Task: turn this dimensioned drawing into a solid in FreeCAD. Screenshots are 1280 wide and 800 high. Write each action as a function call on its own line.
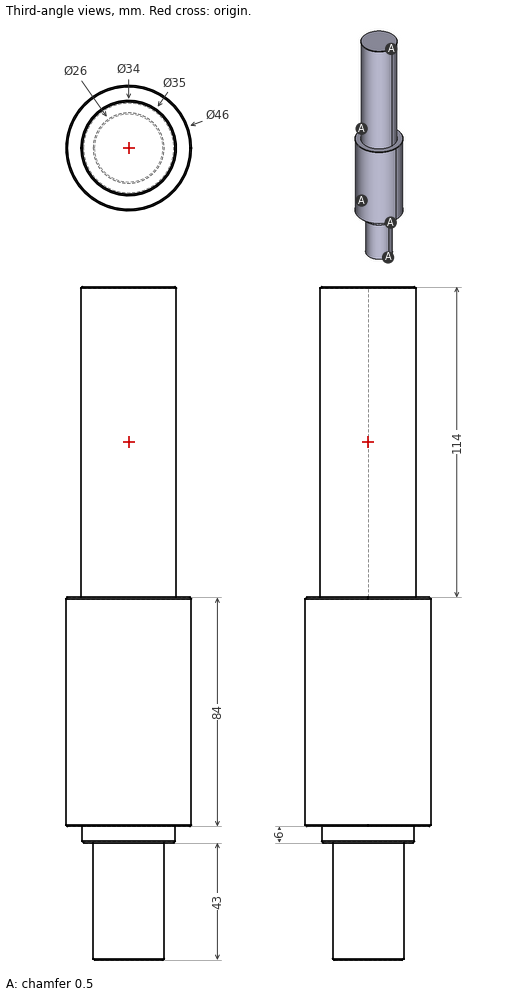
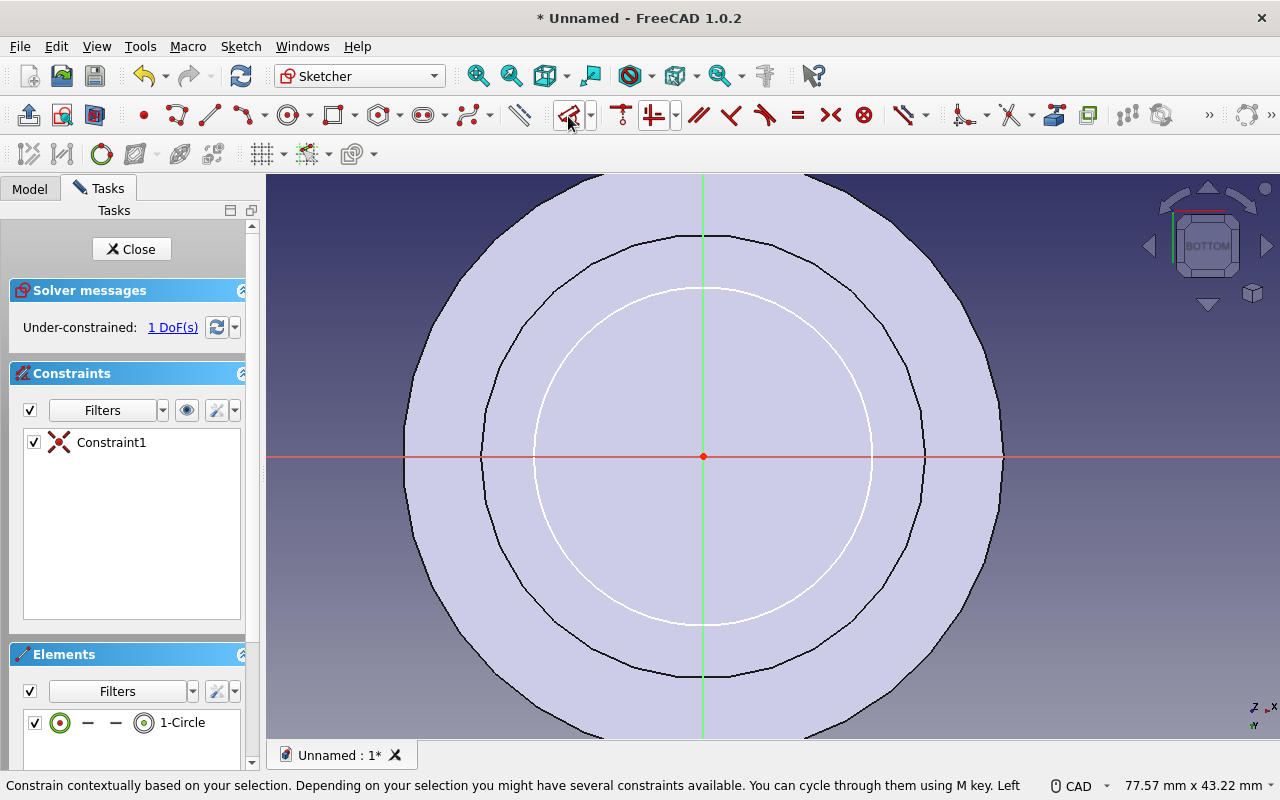
click(822, 336)
click(844, 313)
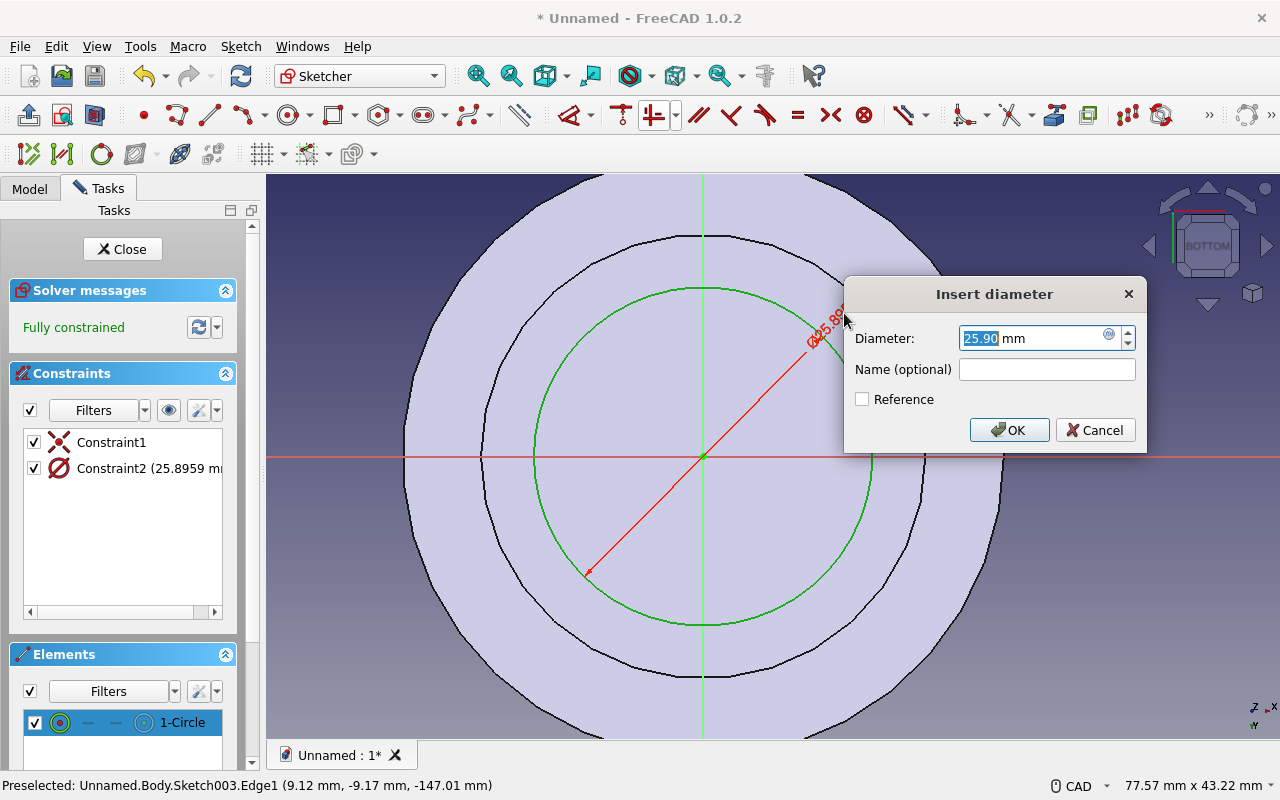
text(26)
key(Return)
key(Escape)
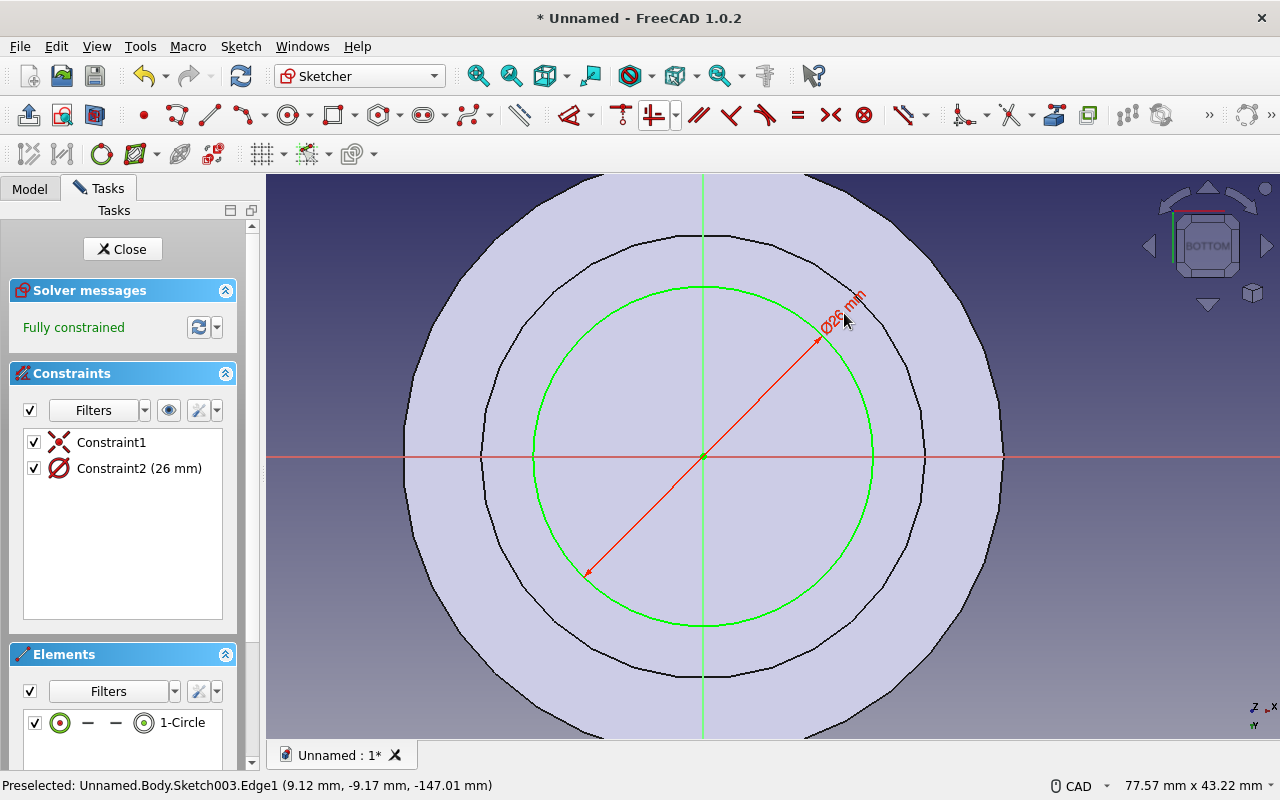
click(123, 249)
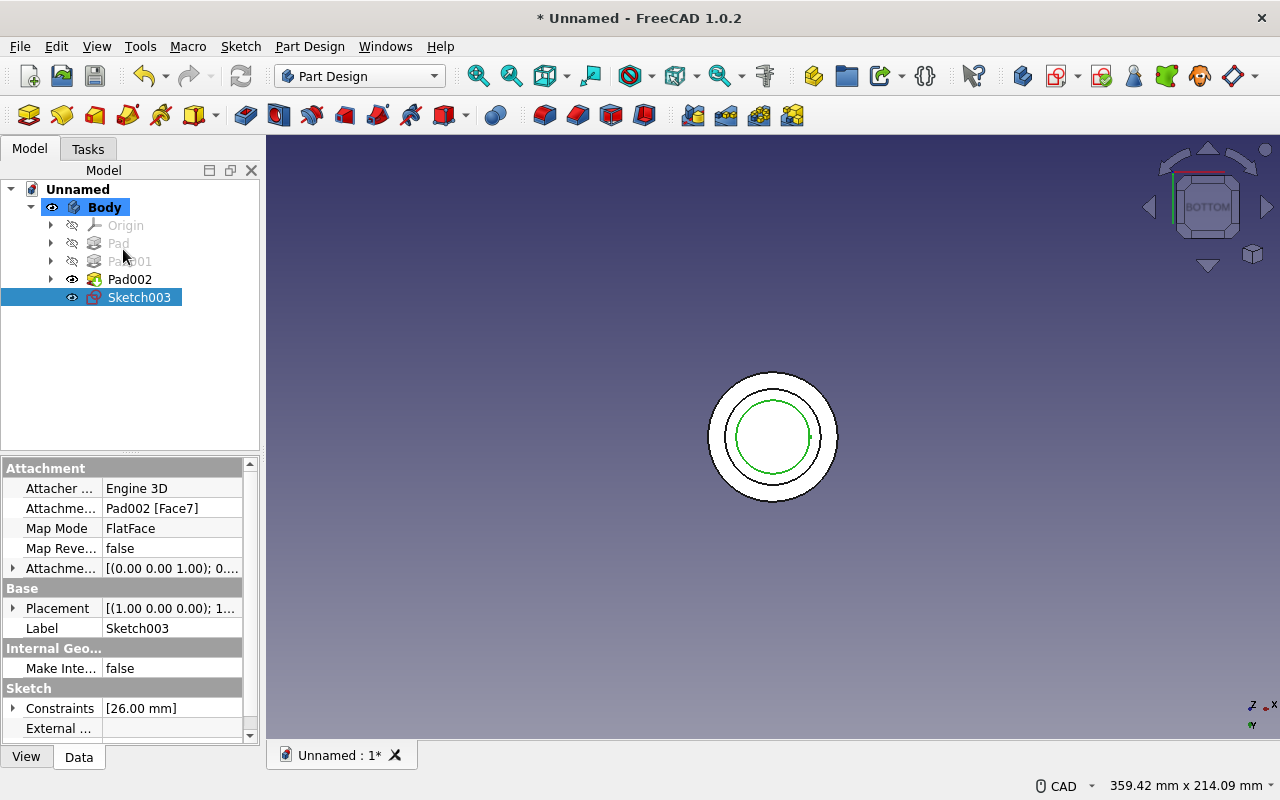
click(29, 116)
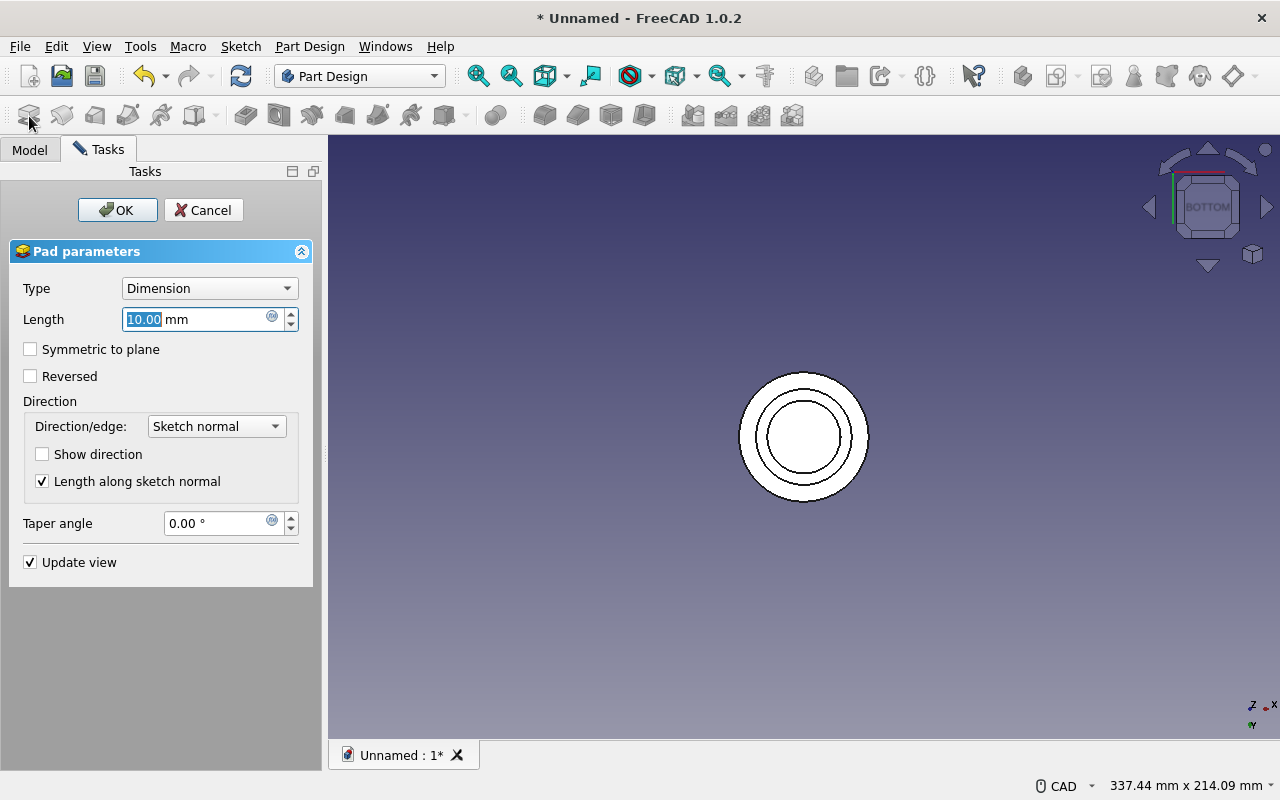
text(43)
key(Tab)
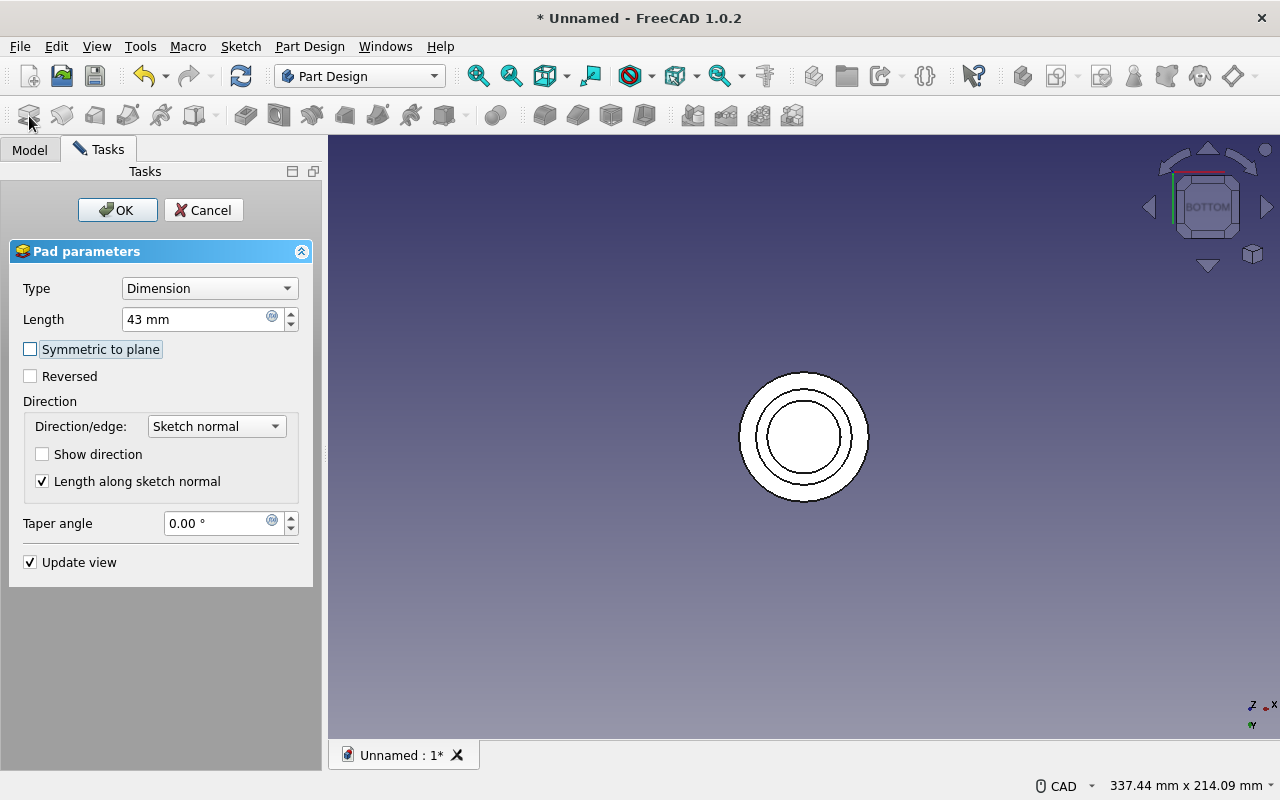
click(118, 210)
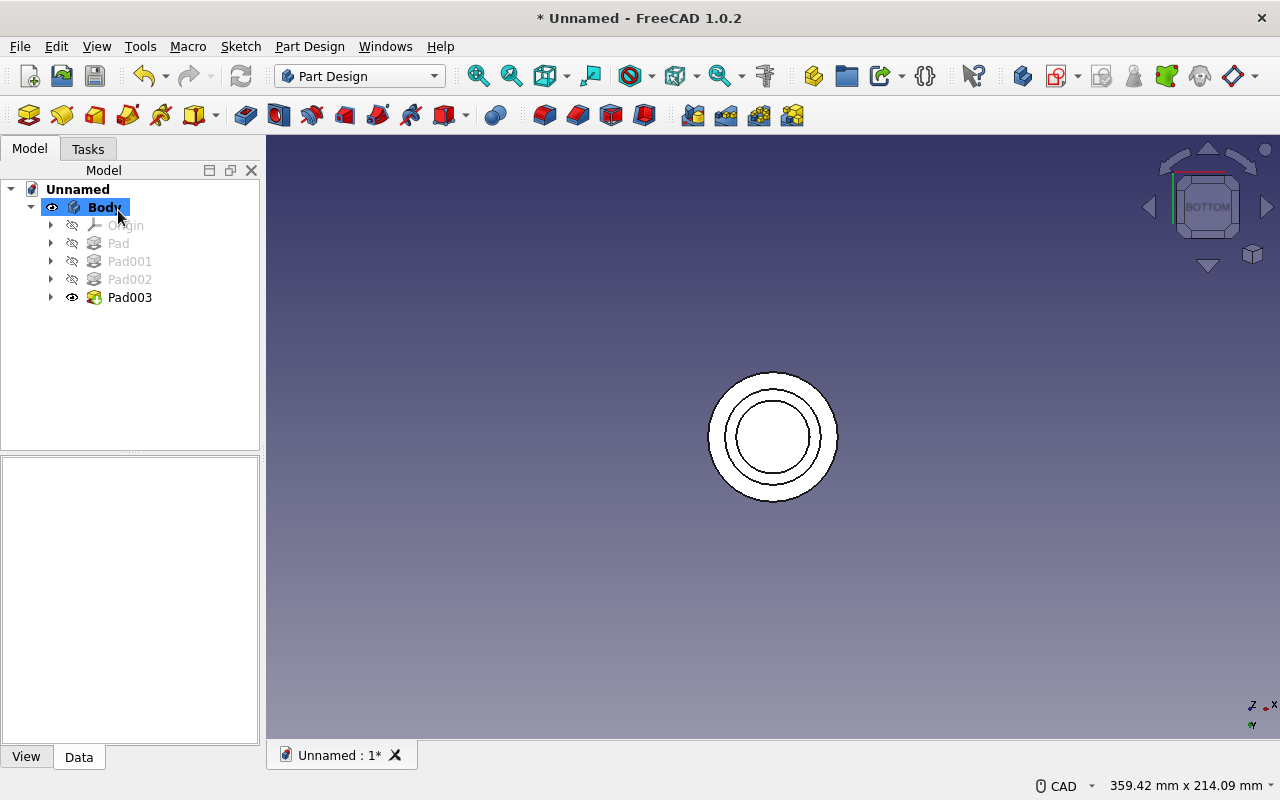
key(v)
key(f)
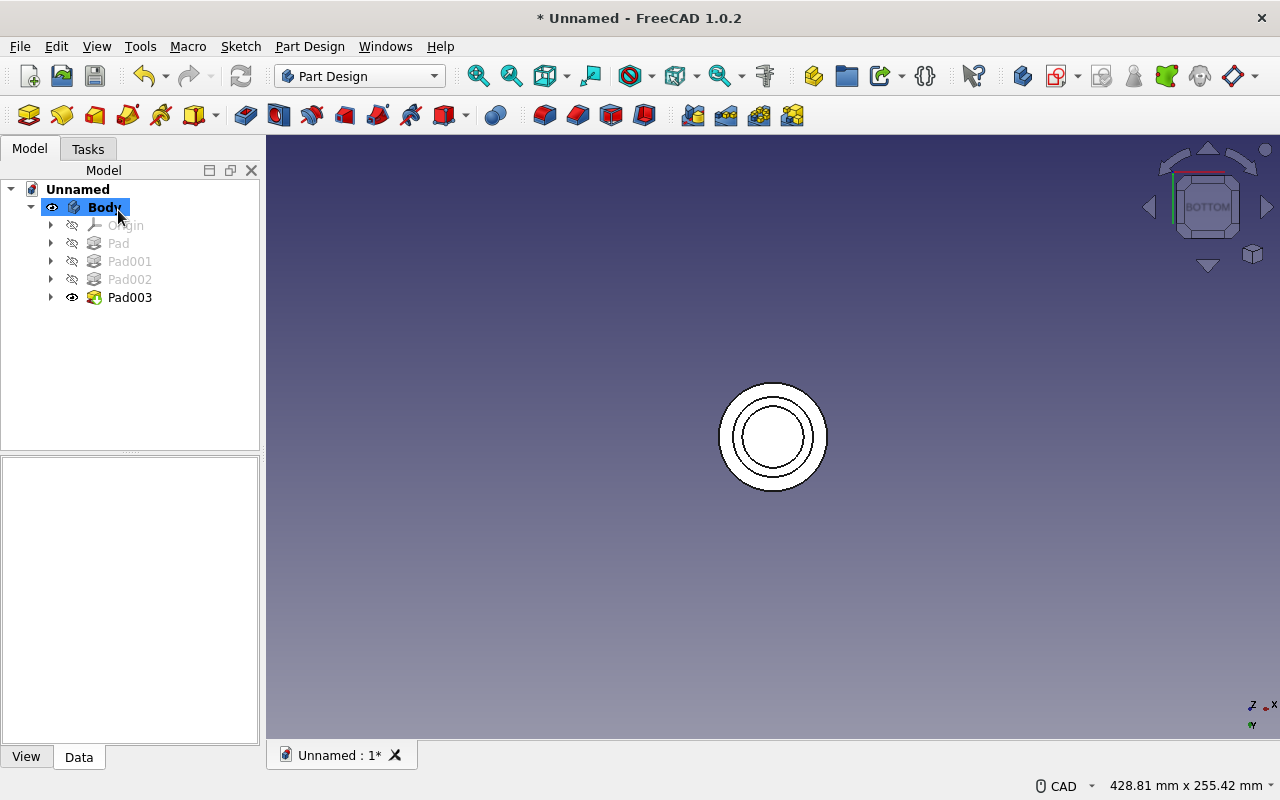
click(733, 436)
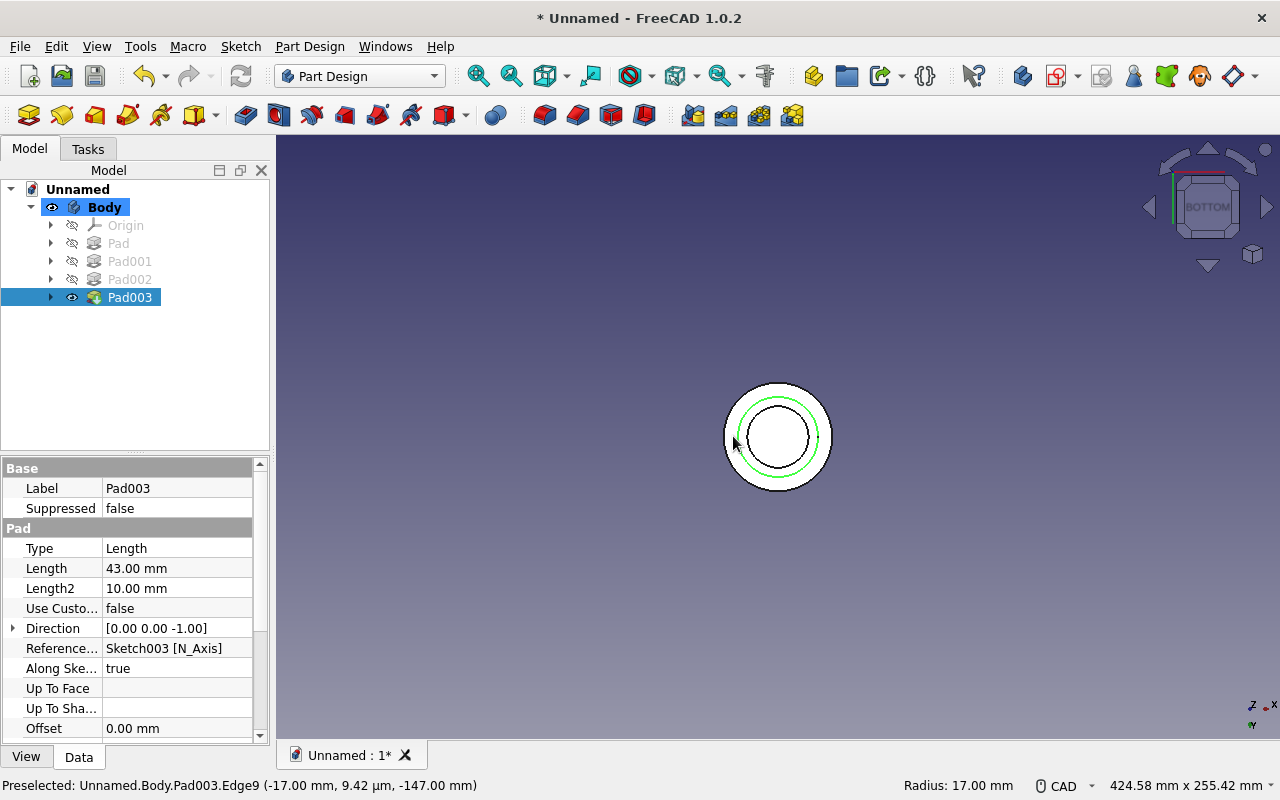
click(747, 436, ctrl)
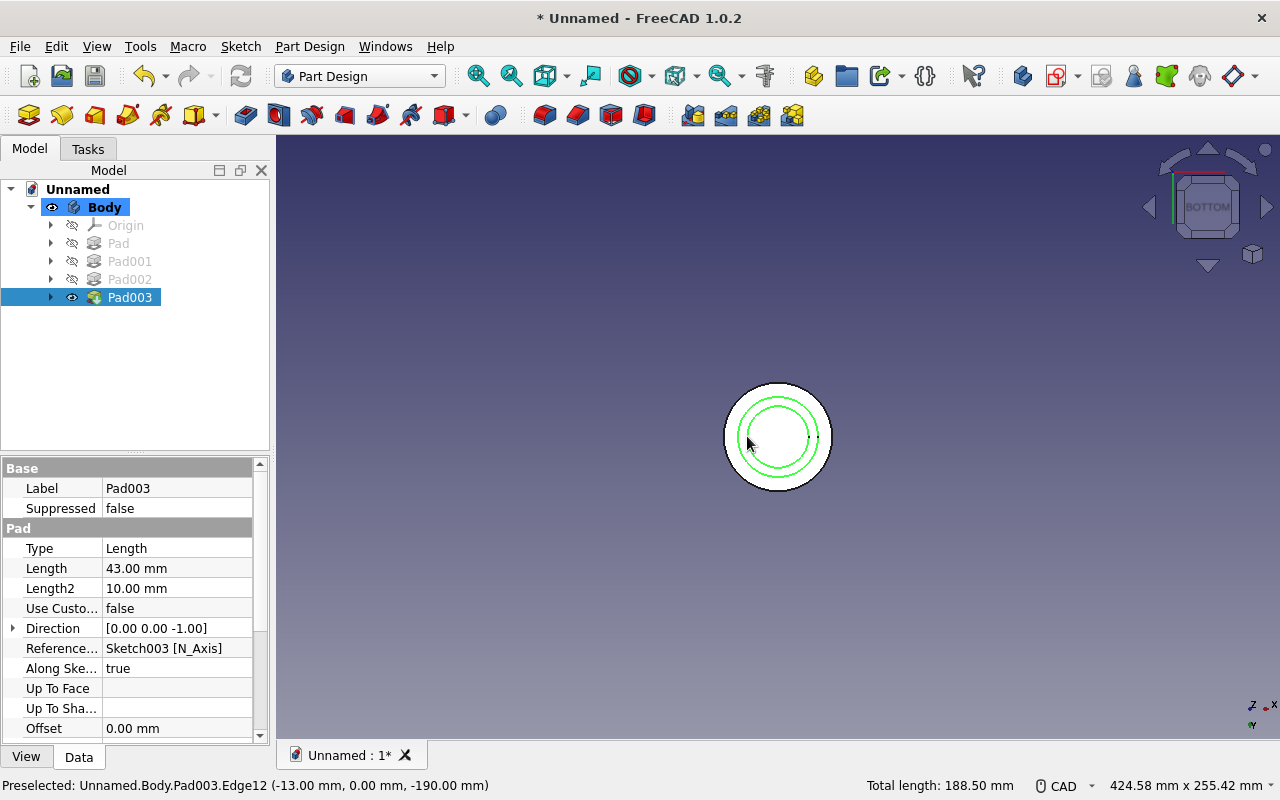
click(724, 436, ctrl)